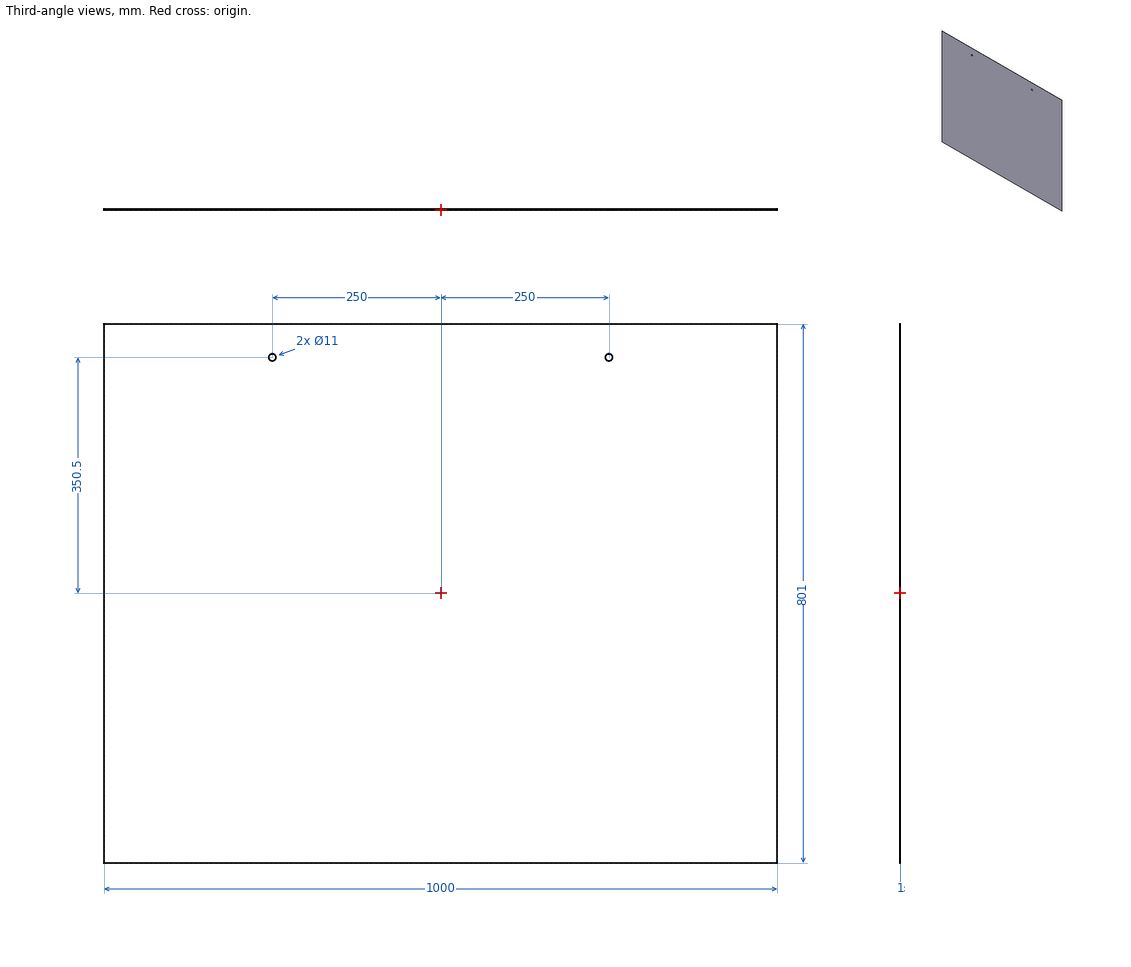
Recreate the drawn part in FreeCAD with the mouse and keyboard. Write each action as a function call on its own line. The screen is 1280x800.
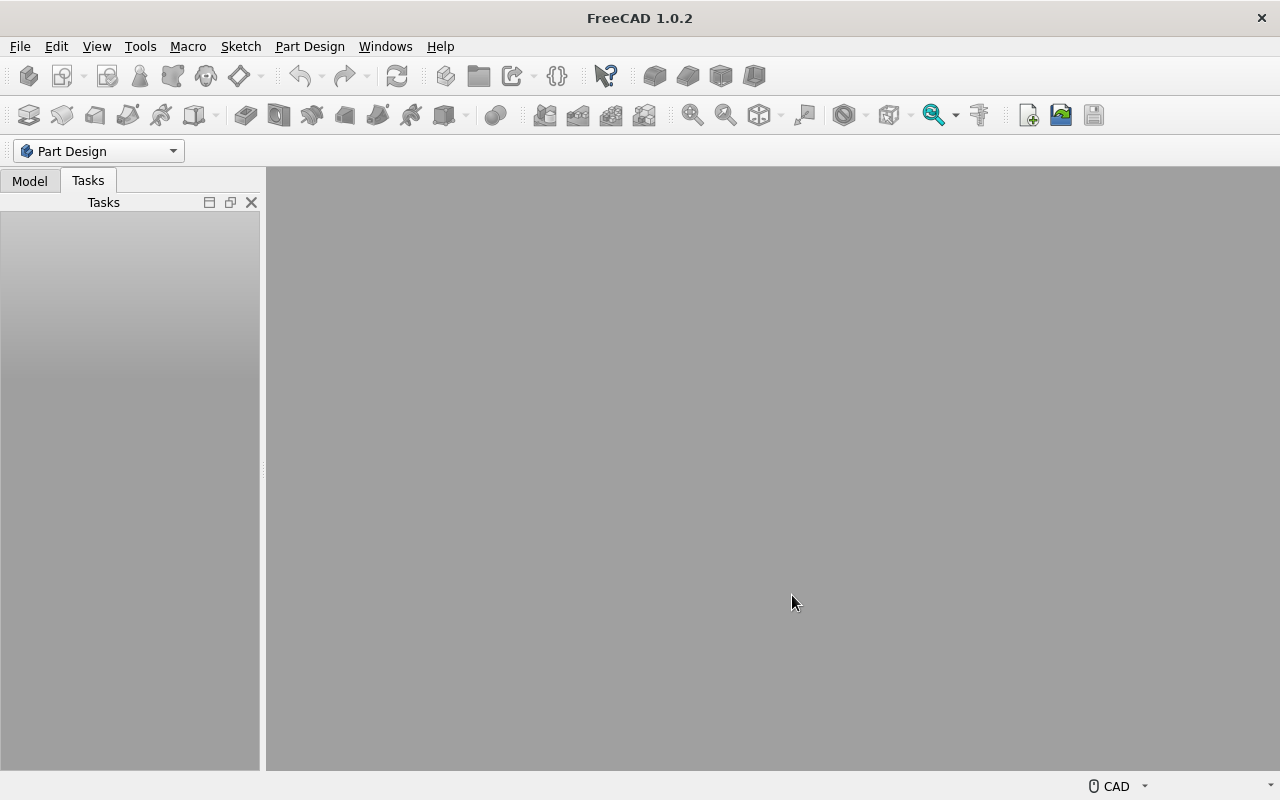
click(1028, 116)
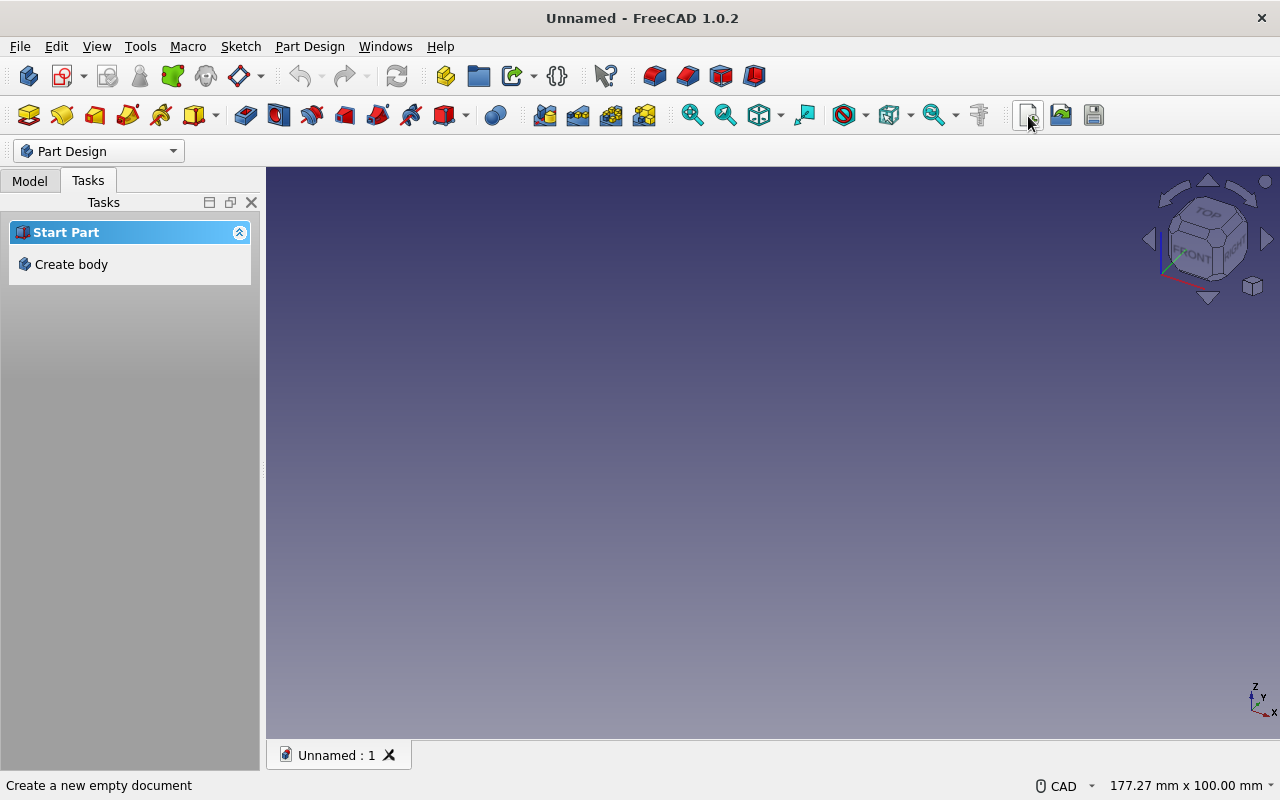
click(62, 76)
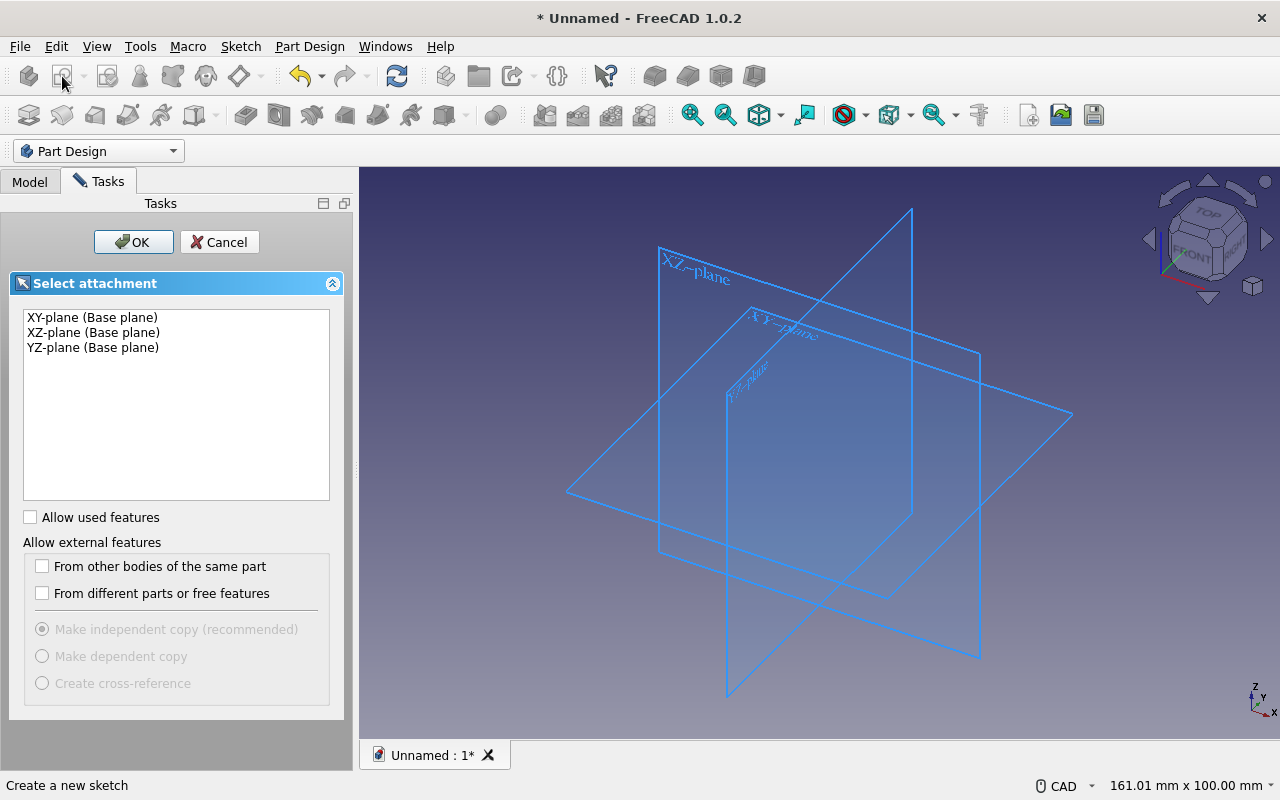
click(84, 332)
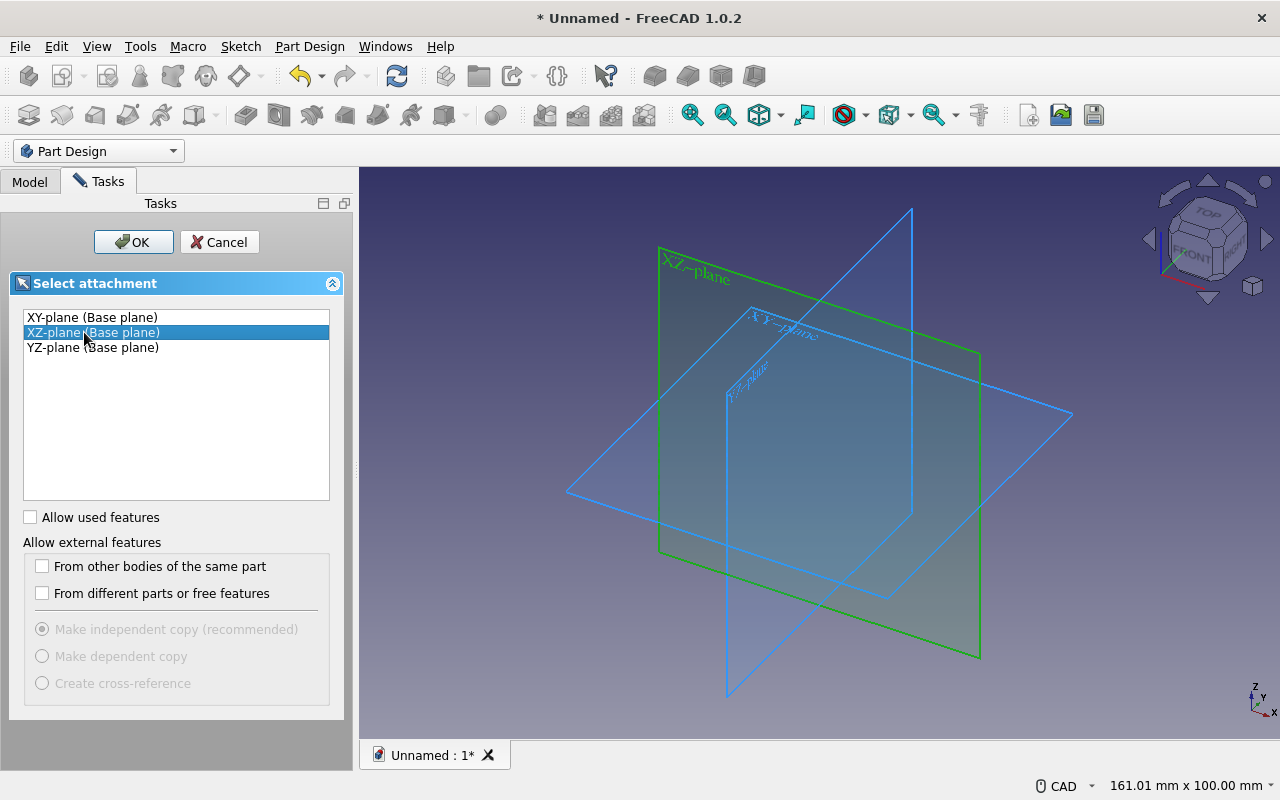
click(134, 242)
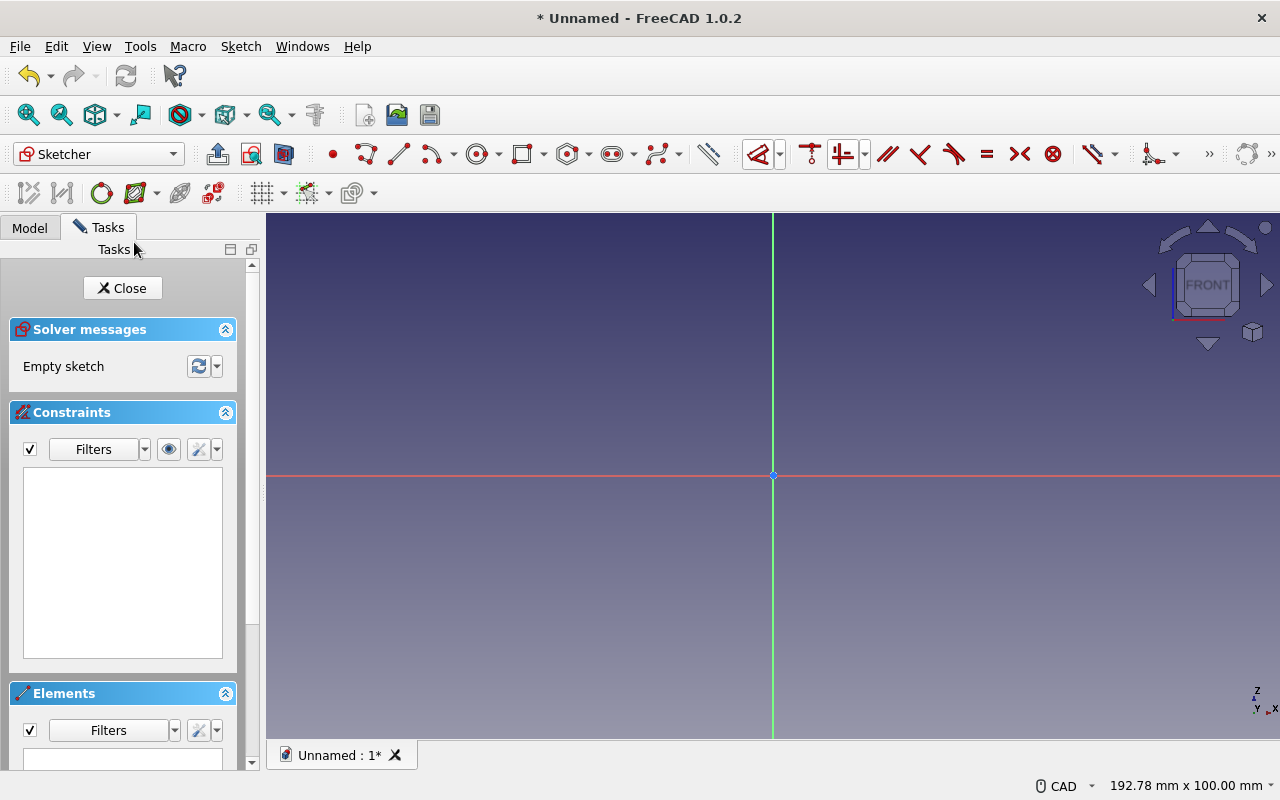
scroll(699, 476, down, 13)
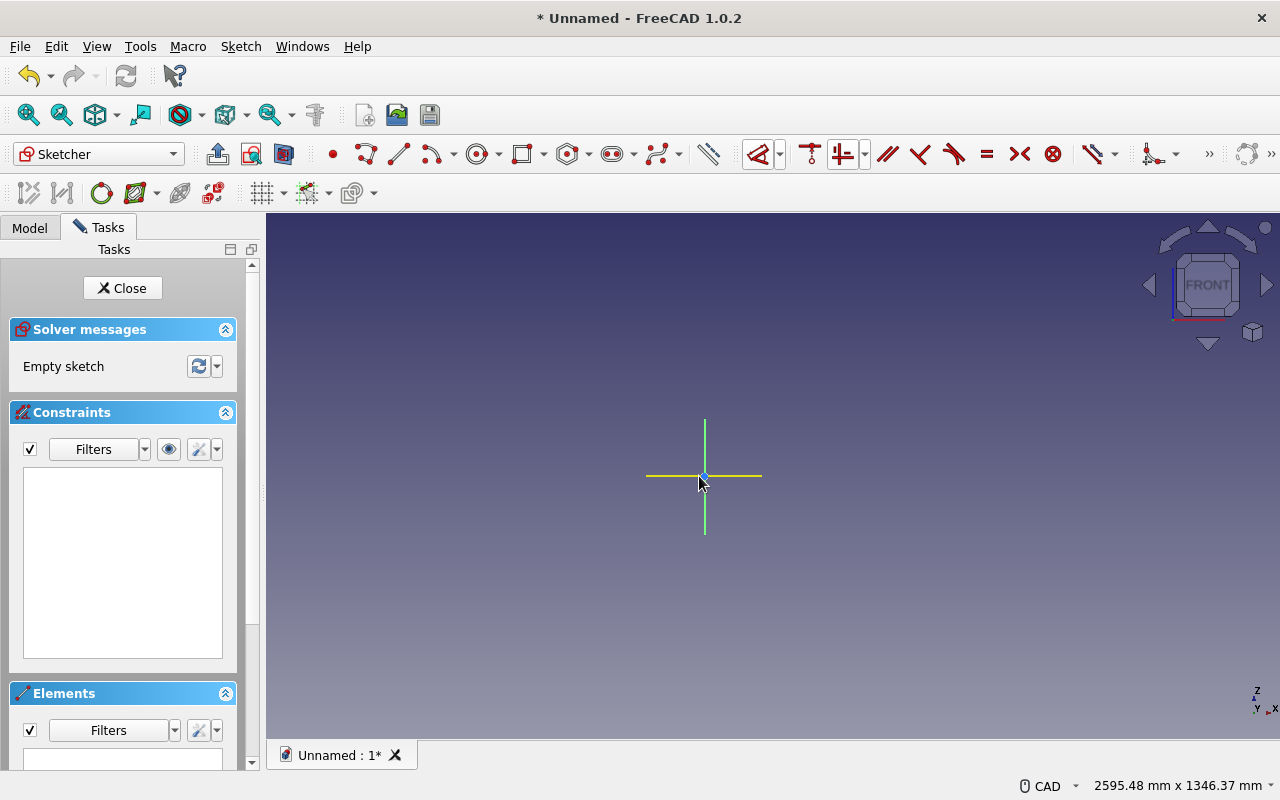
key(g)
key(v)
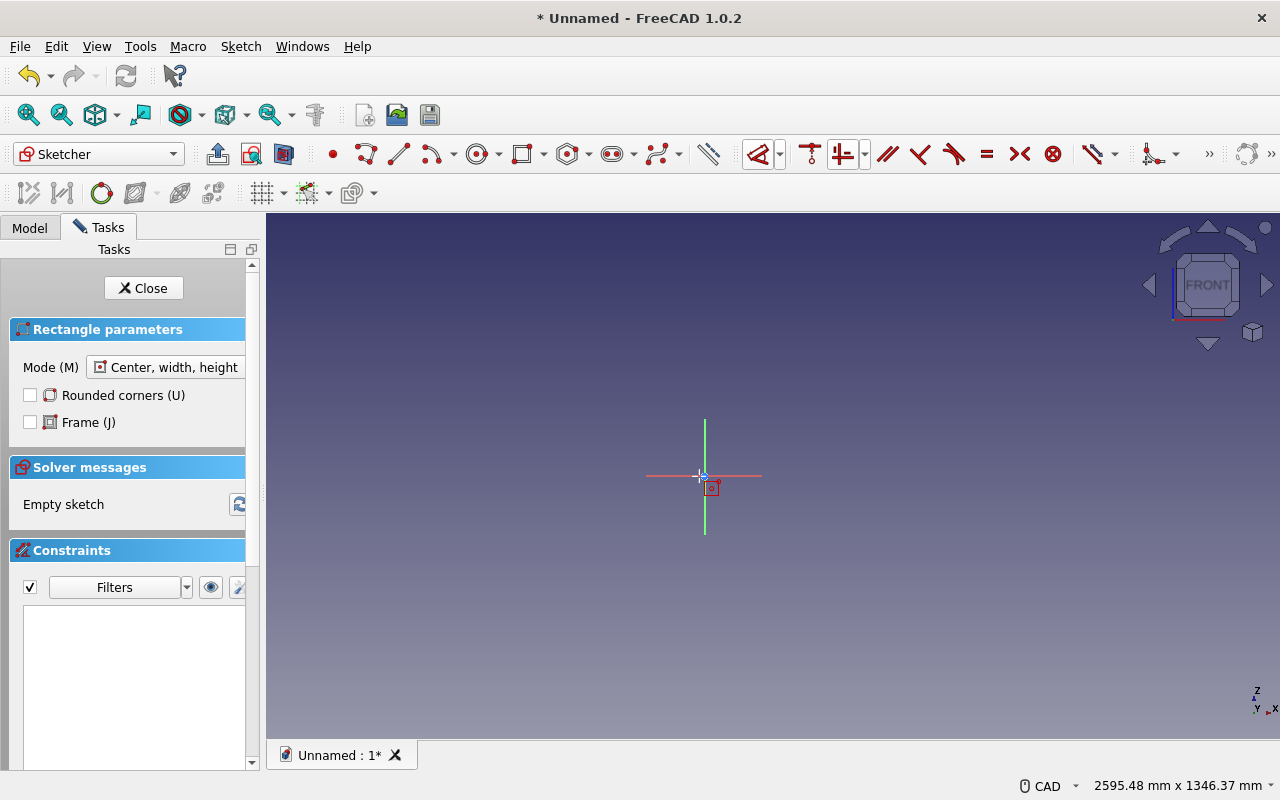
click(705, 476)
move(900, 320)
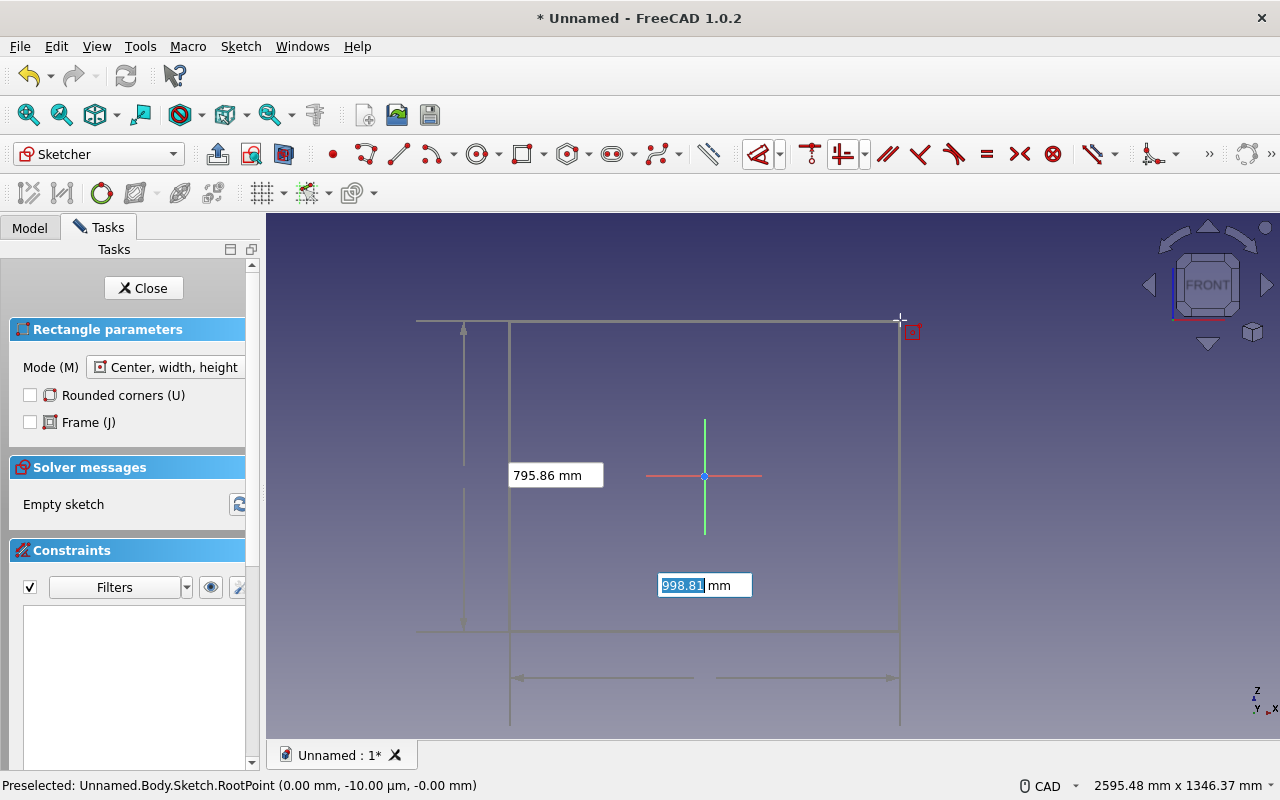
text(1000)
key(Tab)
text(801)
key(Return)
key(Escape)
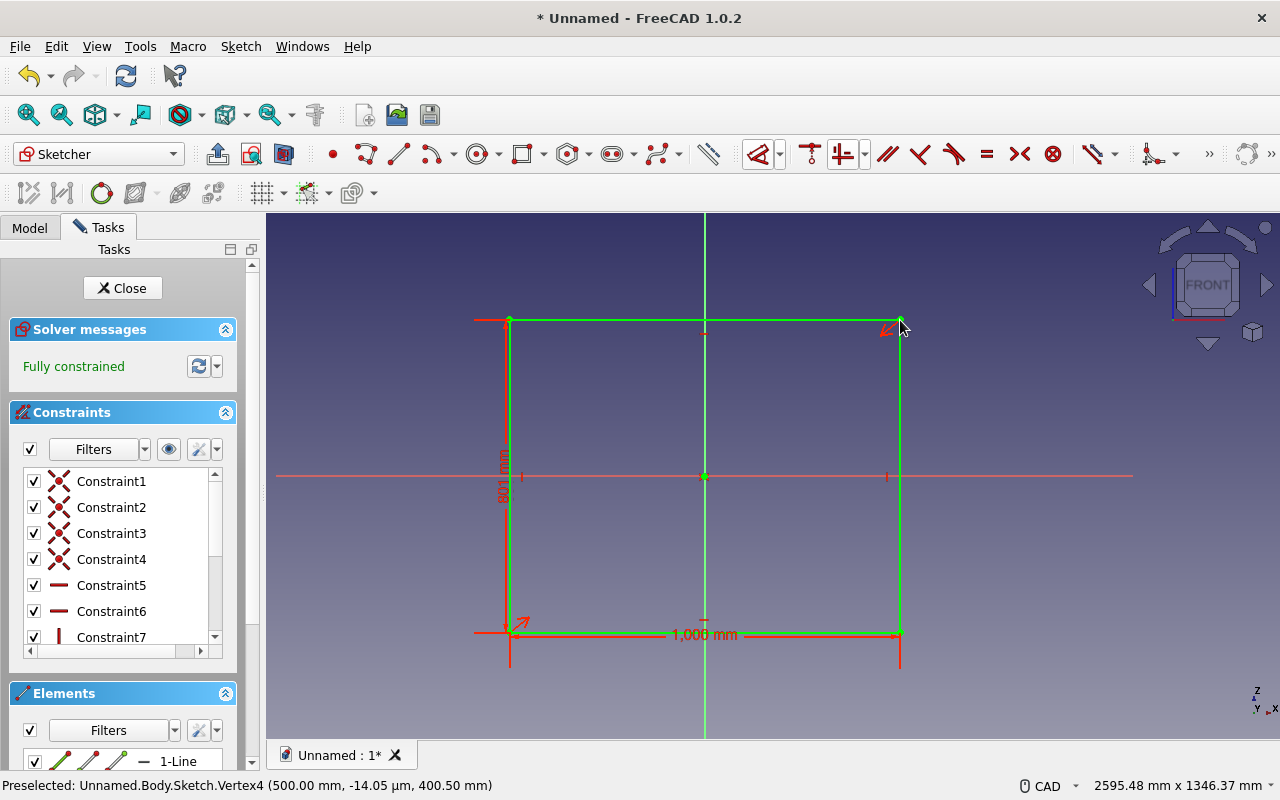
click(123, 288)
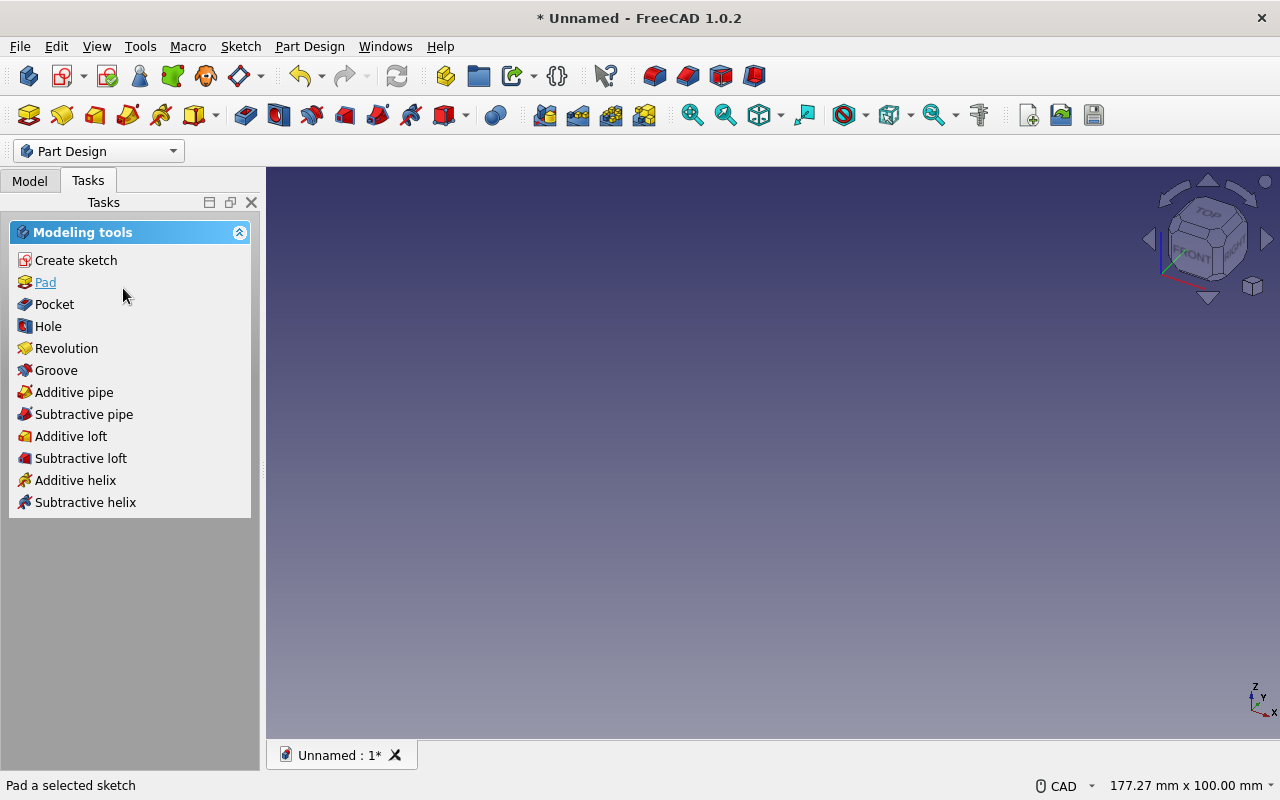
click(29, 116)